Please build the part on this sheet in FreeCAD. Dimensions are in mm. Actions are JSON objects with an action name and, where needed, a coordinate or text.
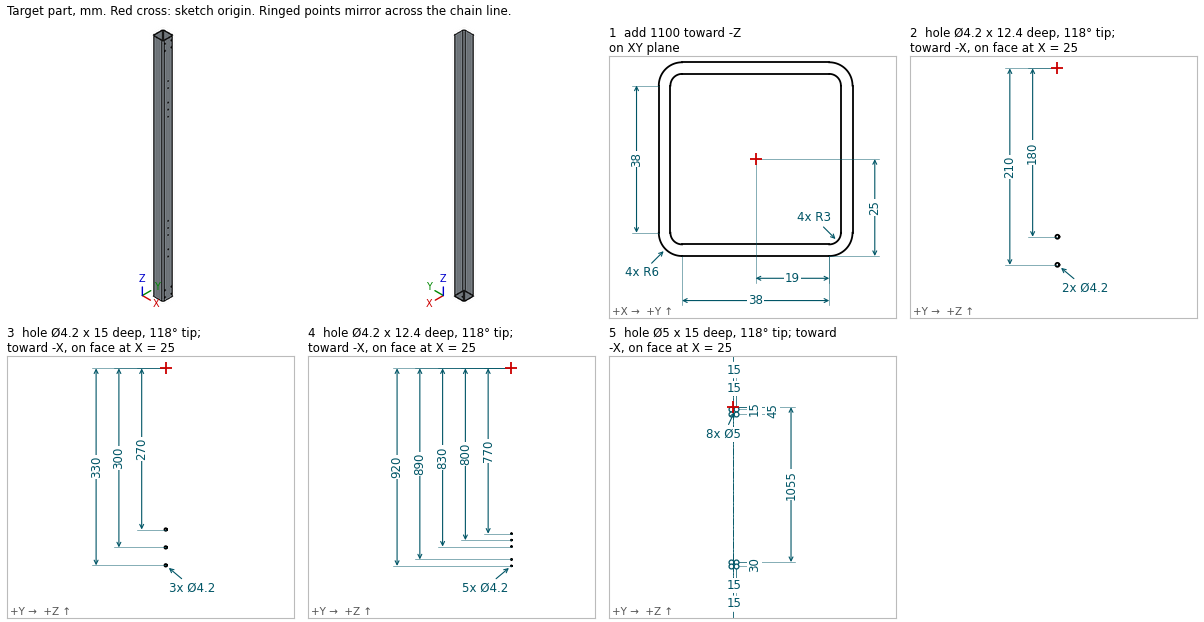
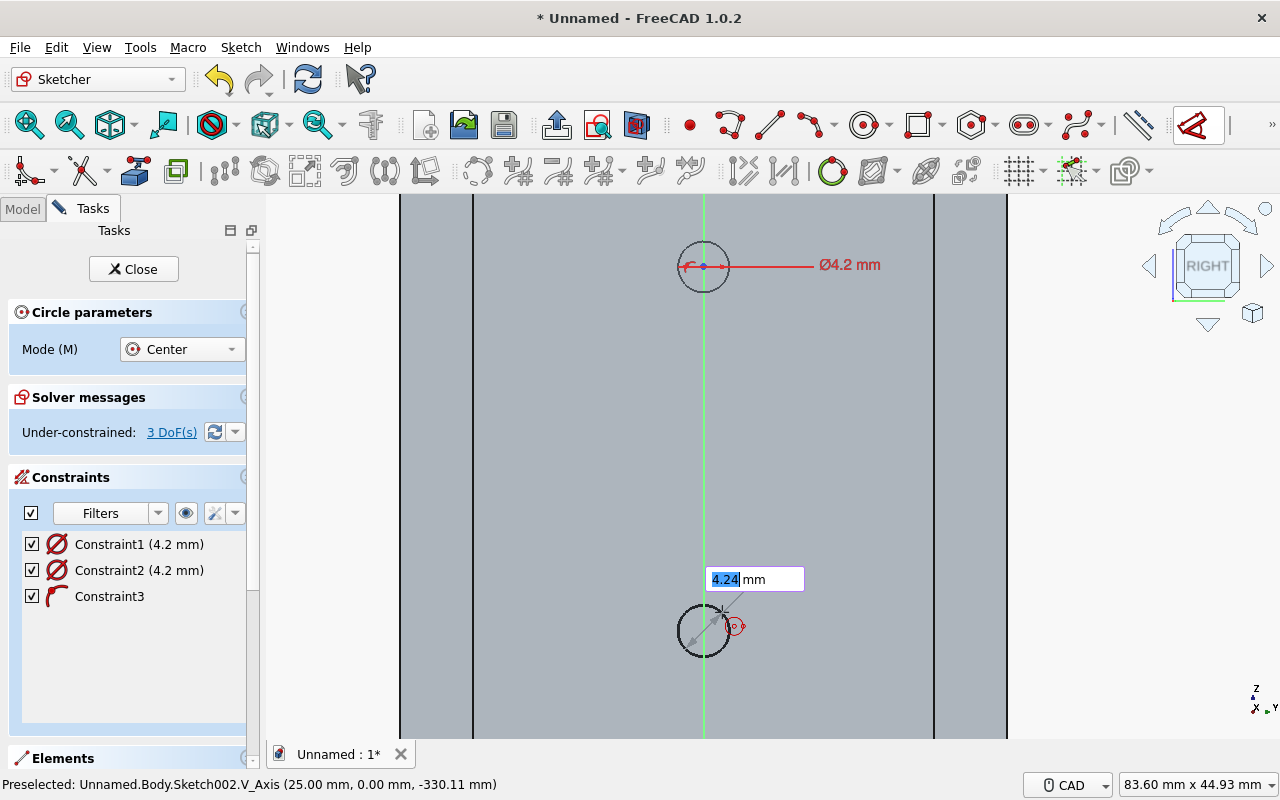
{"action": "type", "text": "4.2"}
{"action": "key", "text": "Return"}
{"action": "key", "text": "Escape"}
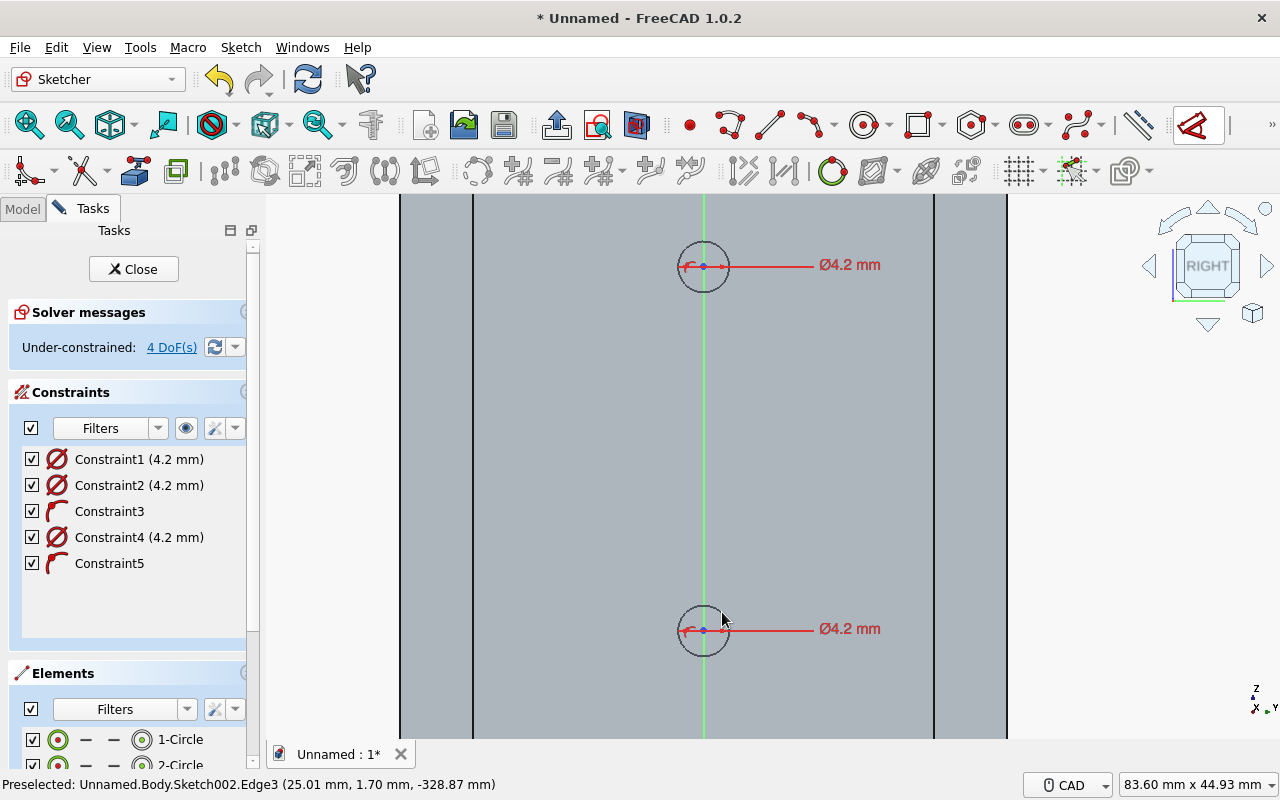
{"action": "scroll", "coordinate": [705, 630], "scroll_direction": "down", "scroll_amount": 4}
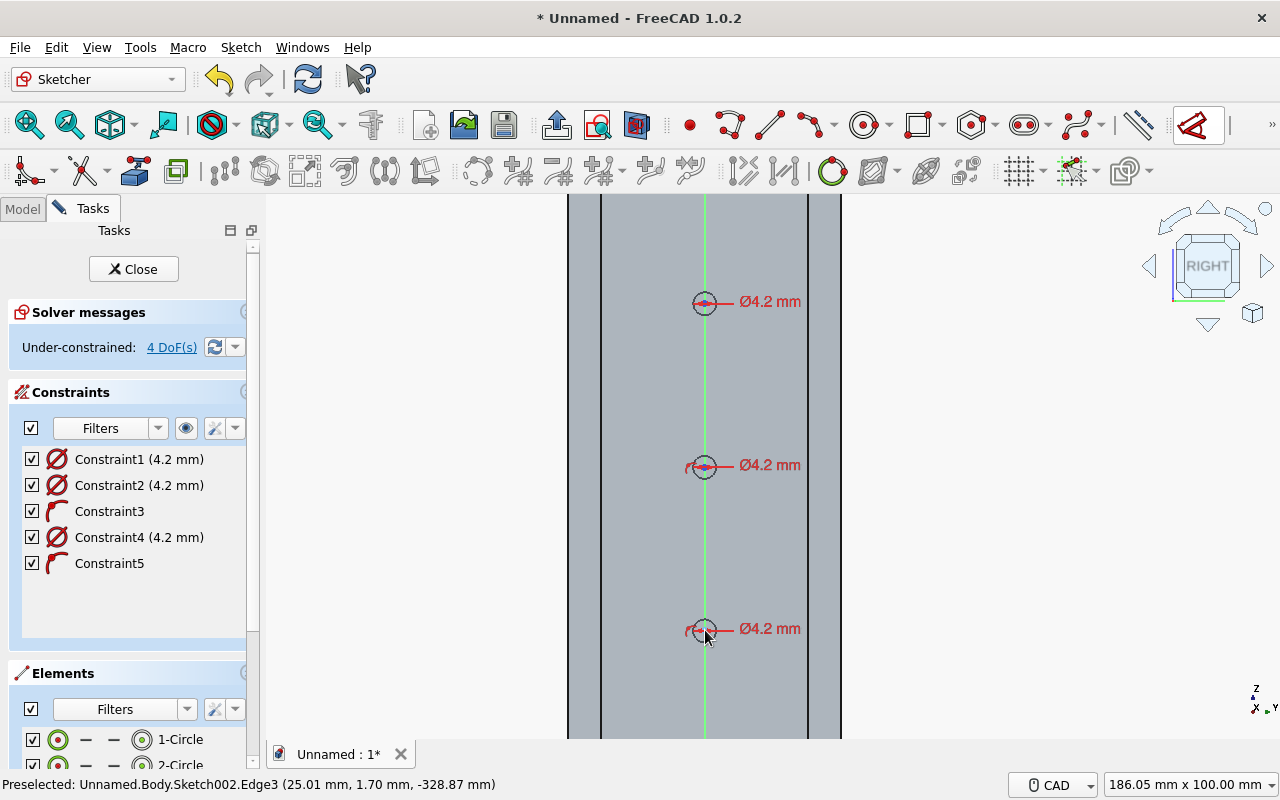
{"action": "left_click", "coordinate": [705, 304]}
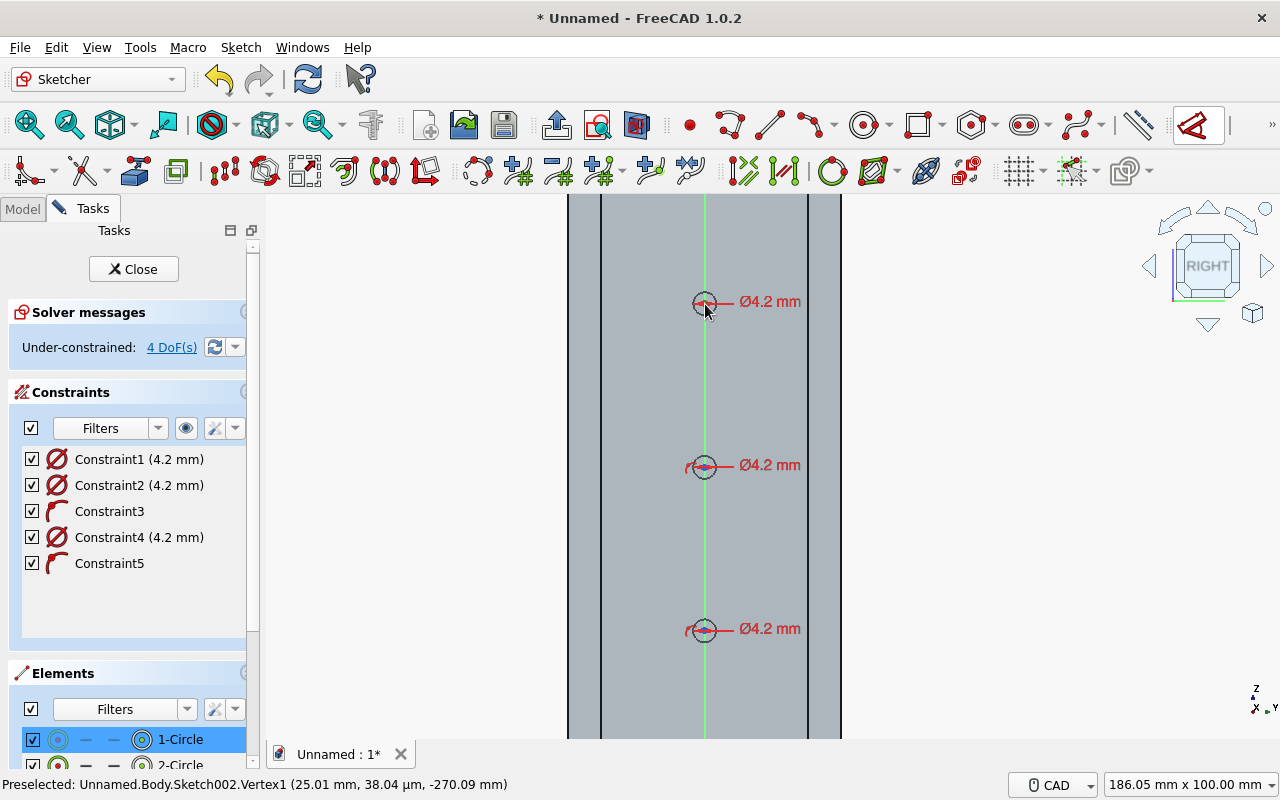
{"action": "left_click", "coordinate": [705, 676]}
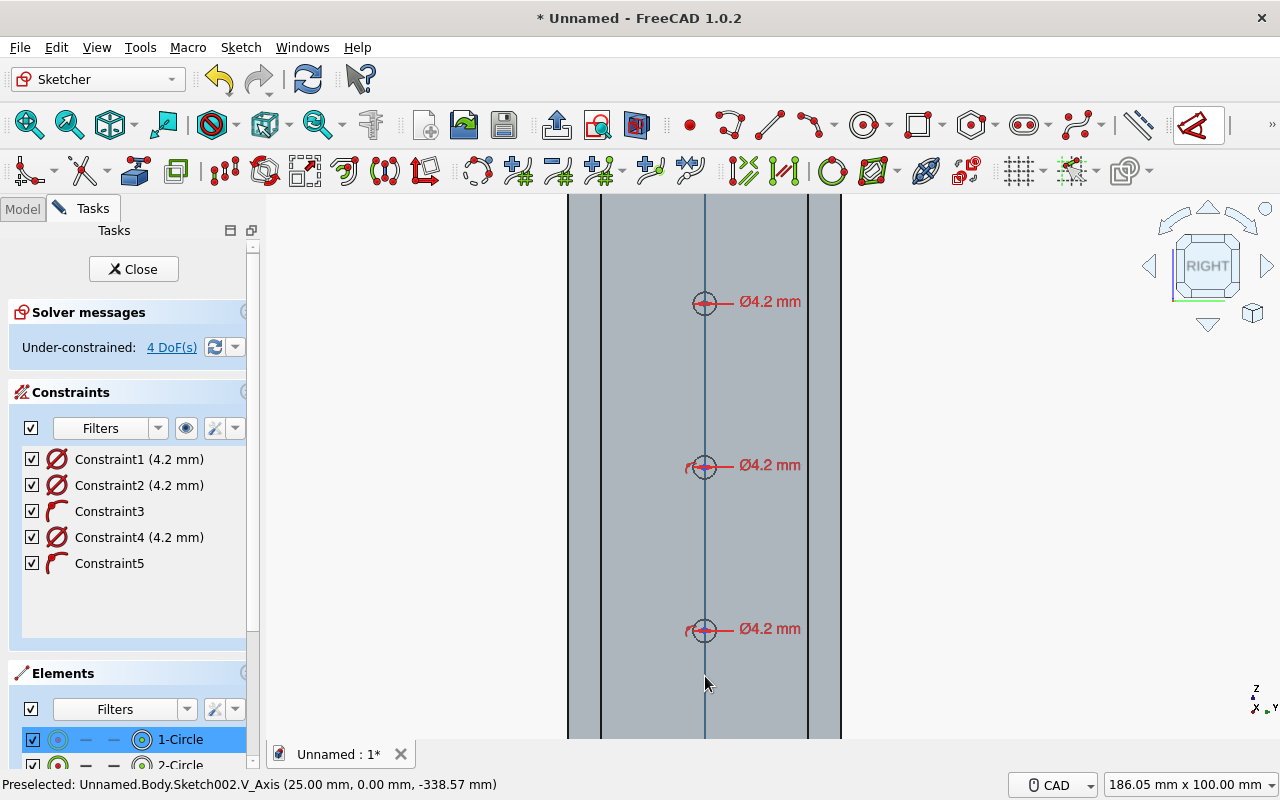
{"action": "key", "text": "c"}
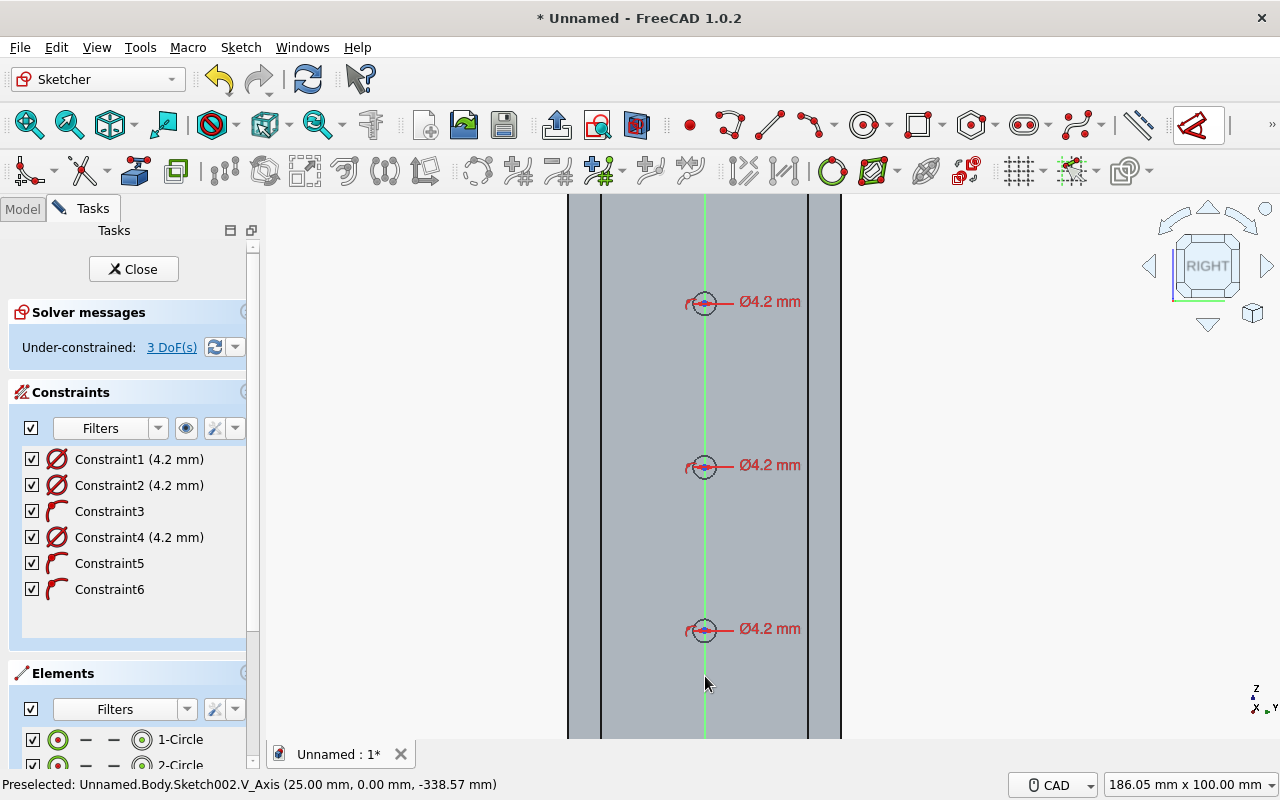
{"action": "left_click", "coordinate": [705, 304]}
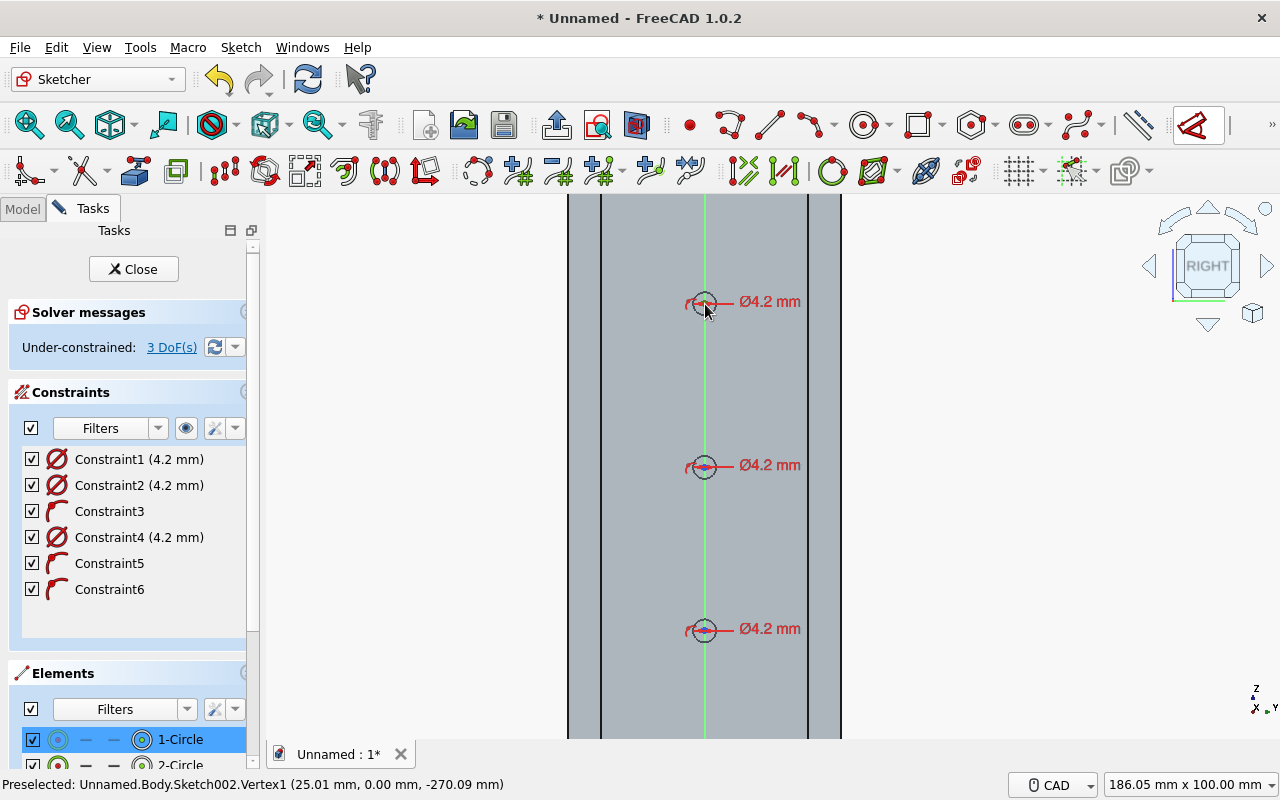
{"action": "left_click", "coordinate": [1218, 126]}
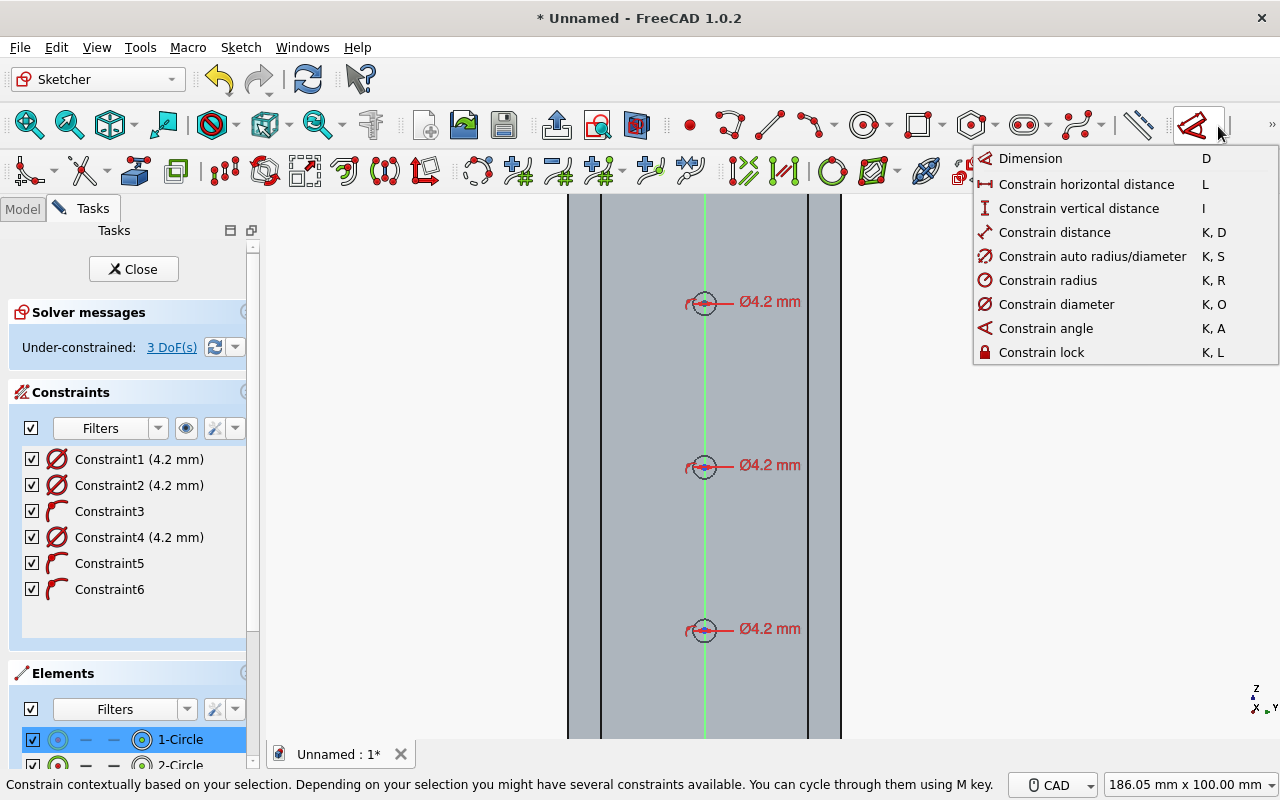
{"action": "left_click", "coordinate": [1126, 208]}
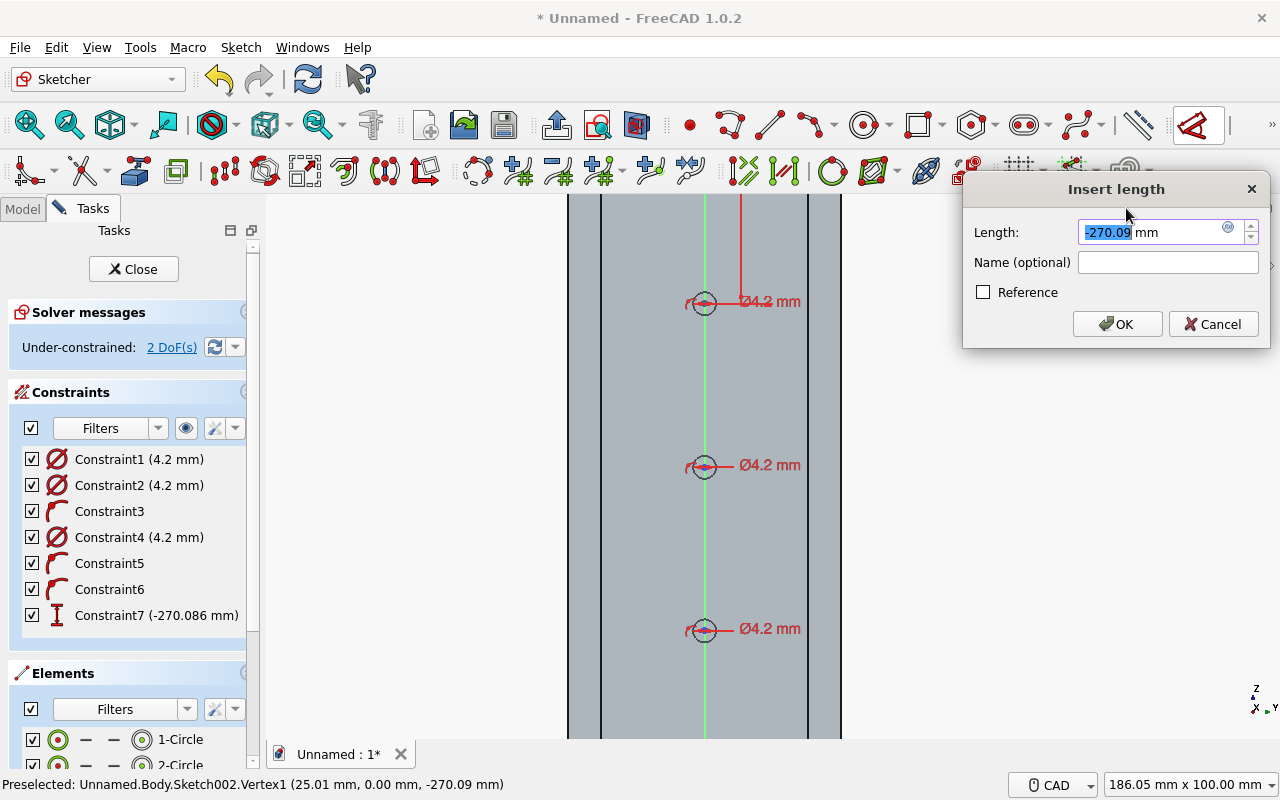
{"action": "type", "text": "-270"}
{"action": "key", "text": "Return"}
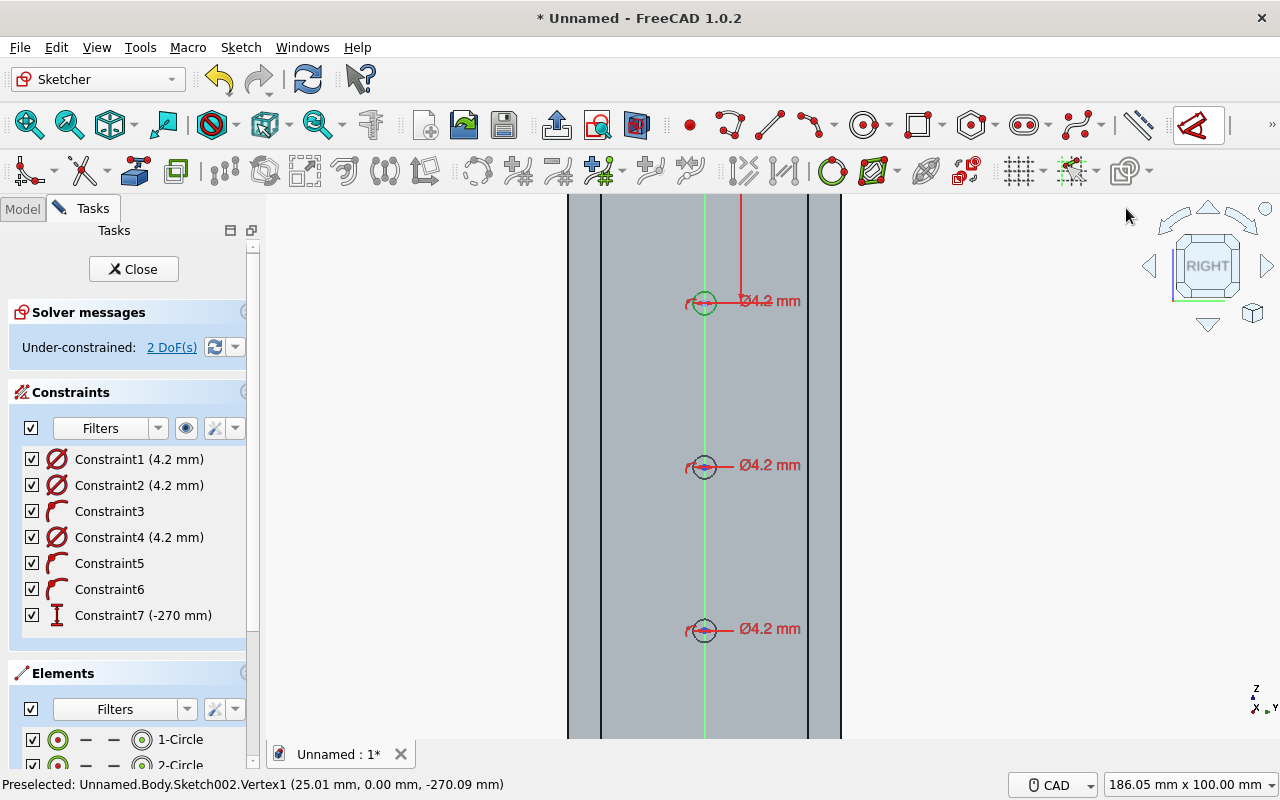
{"action": "left_click", "coordinate": [705, 467]}